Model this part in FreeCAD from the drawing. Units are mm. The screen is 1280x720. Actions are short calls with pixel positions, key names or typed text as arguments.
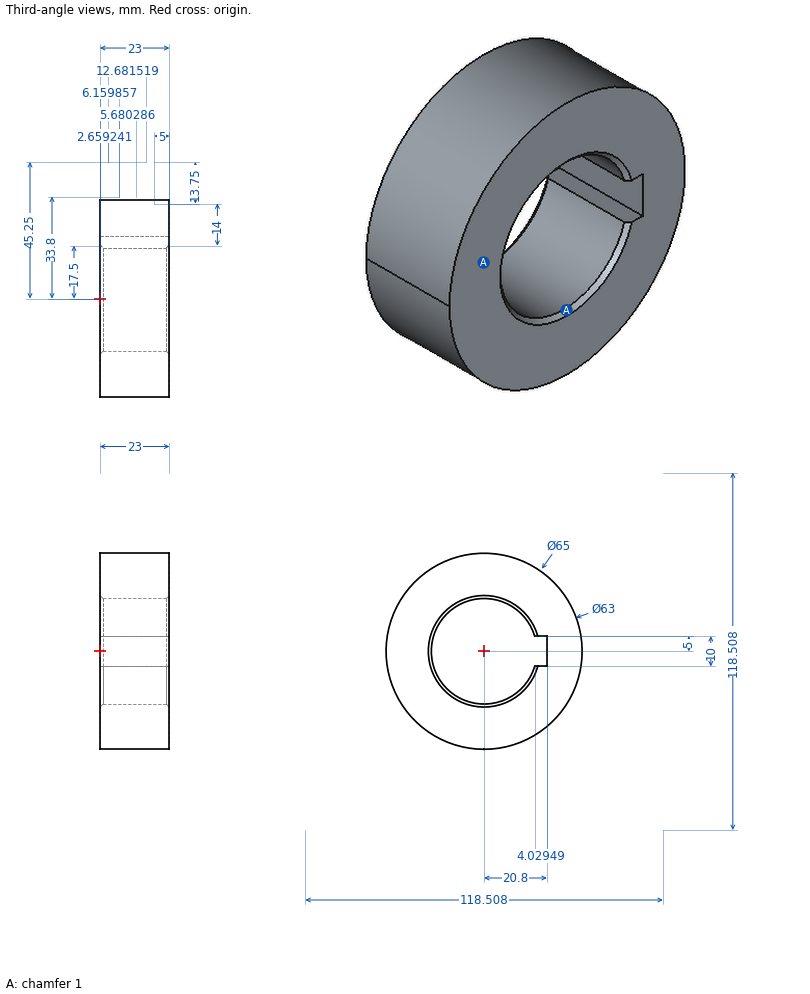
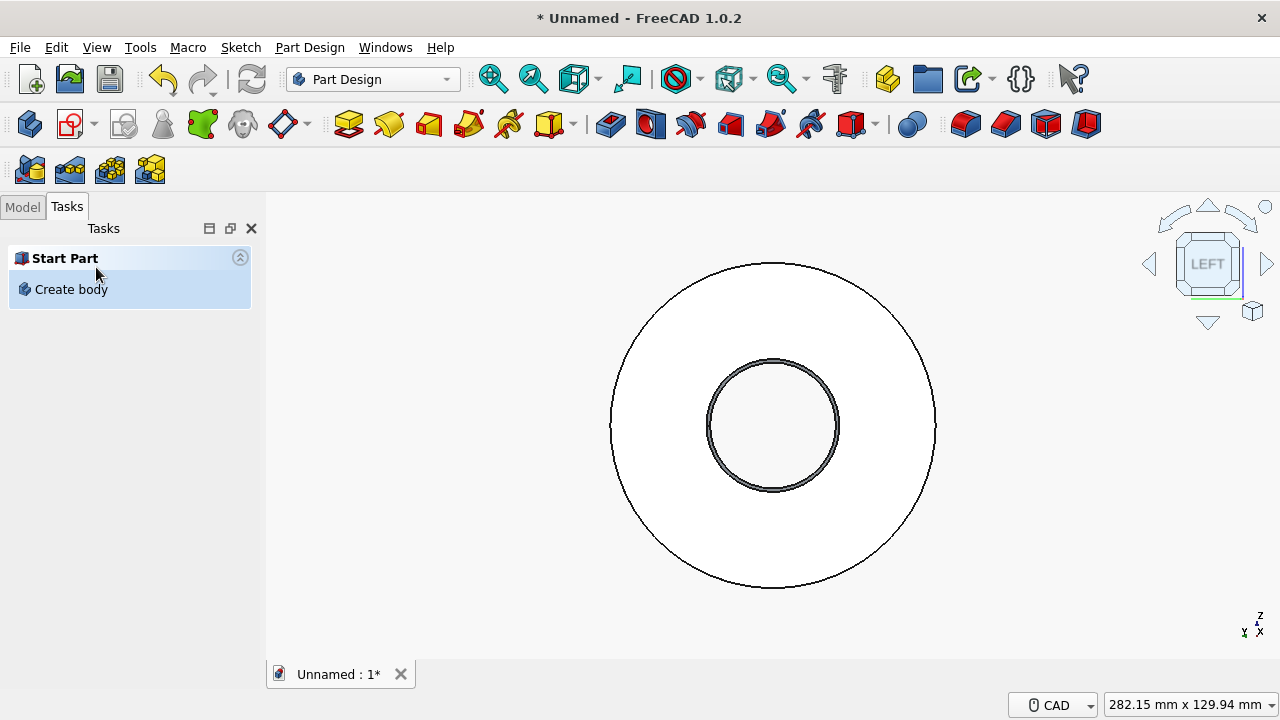
click(70, 124)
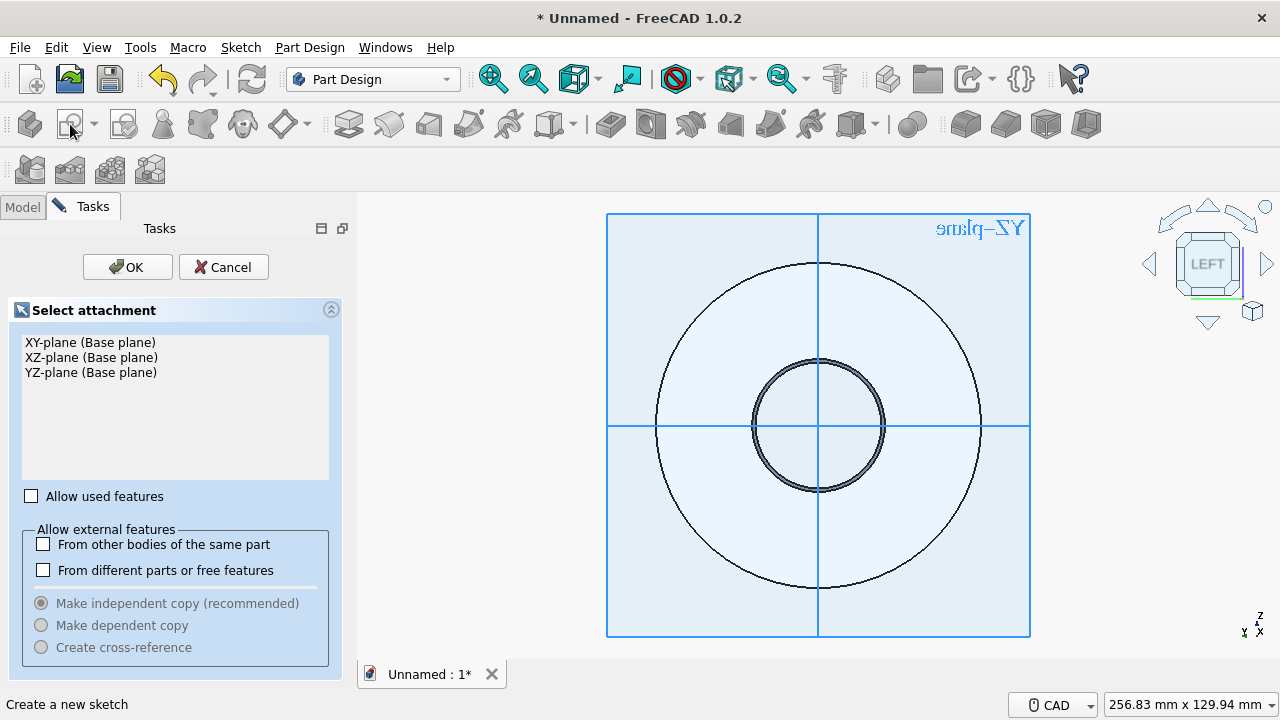
click(82, 372)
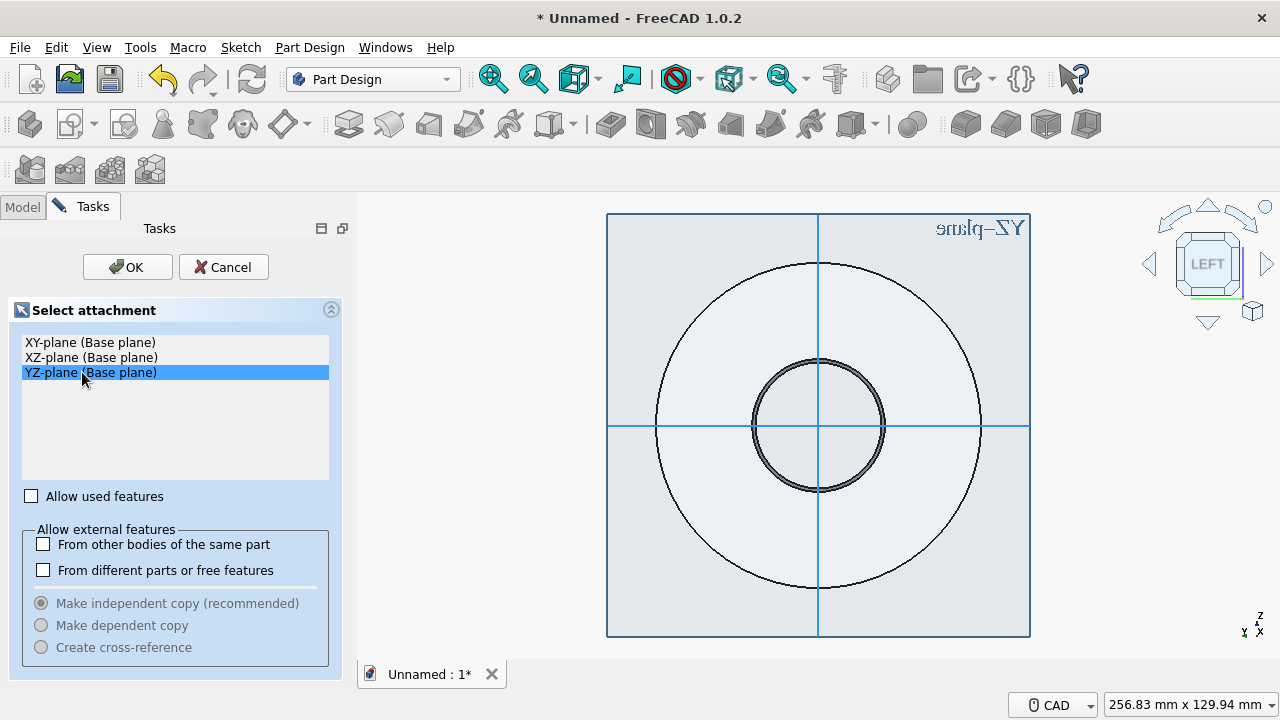
click(128, 267)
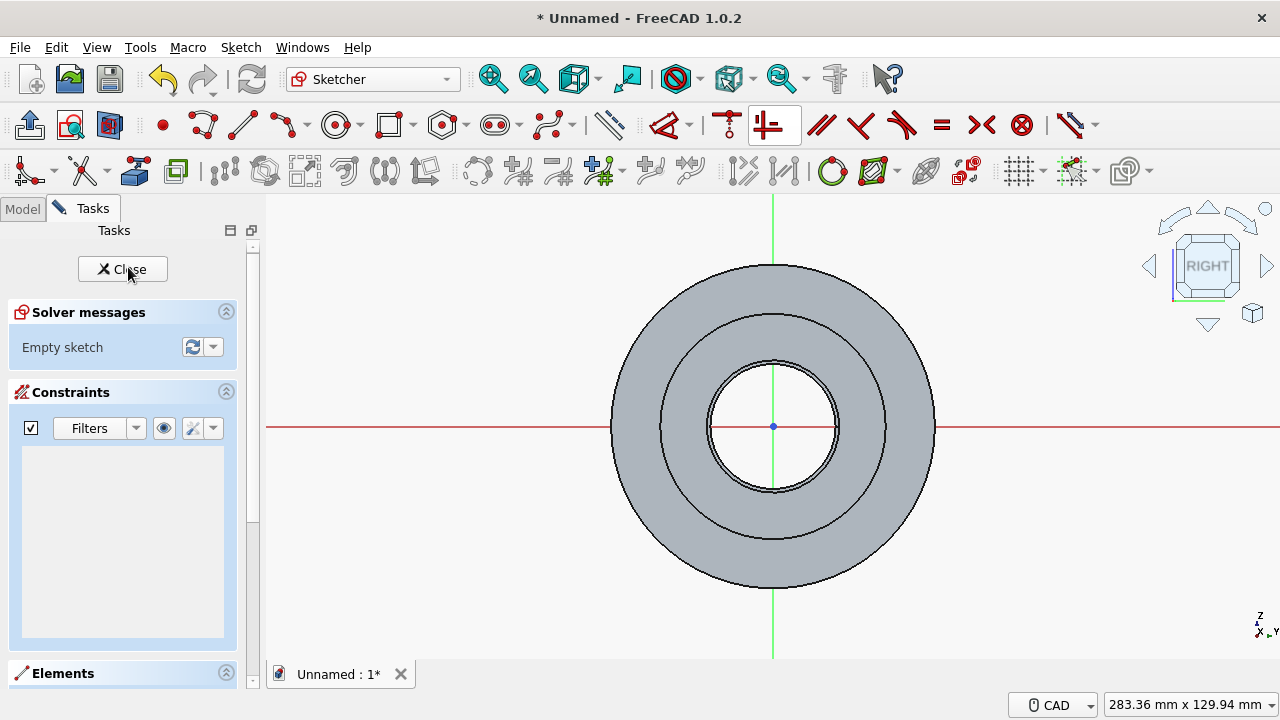
key(q)
key(s)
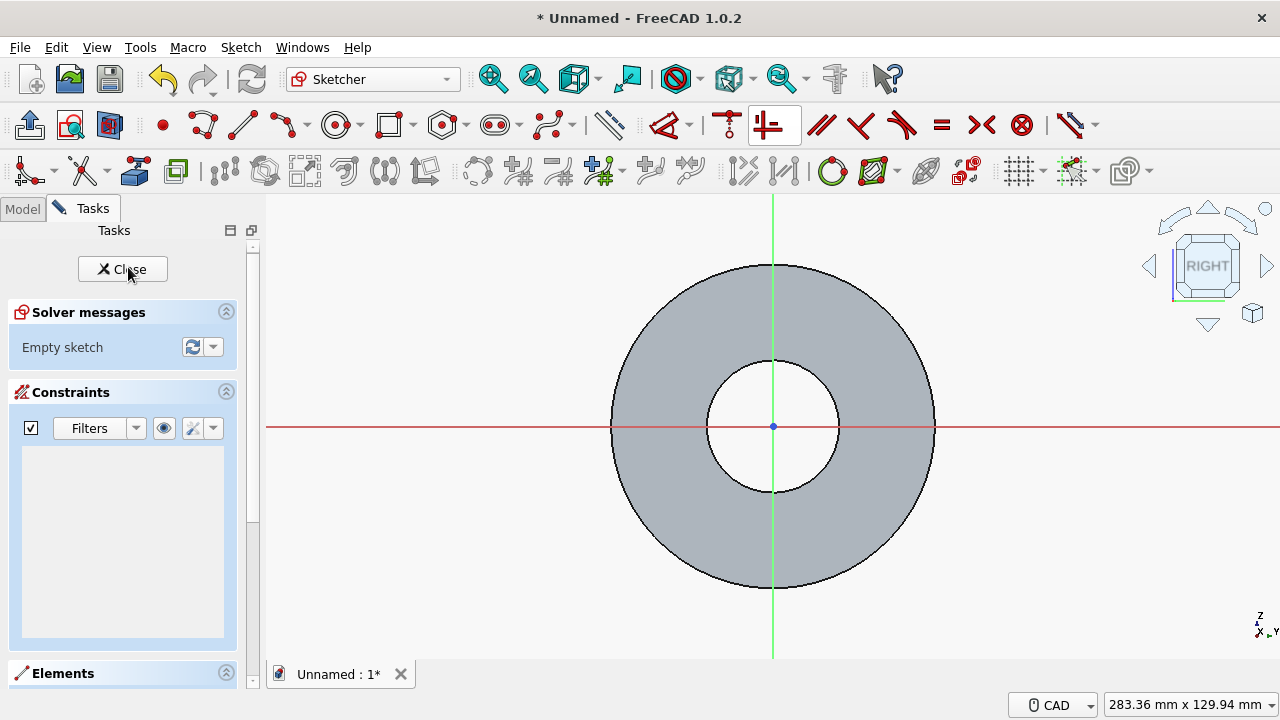
scroll(827, 426, up, 10)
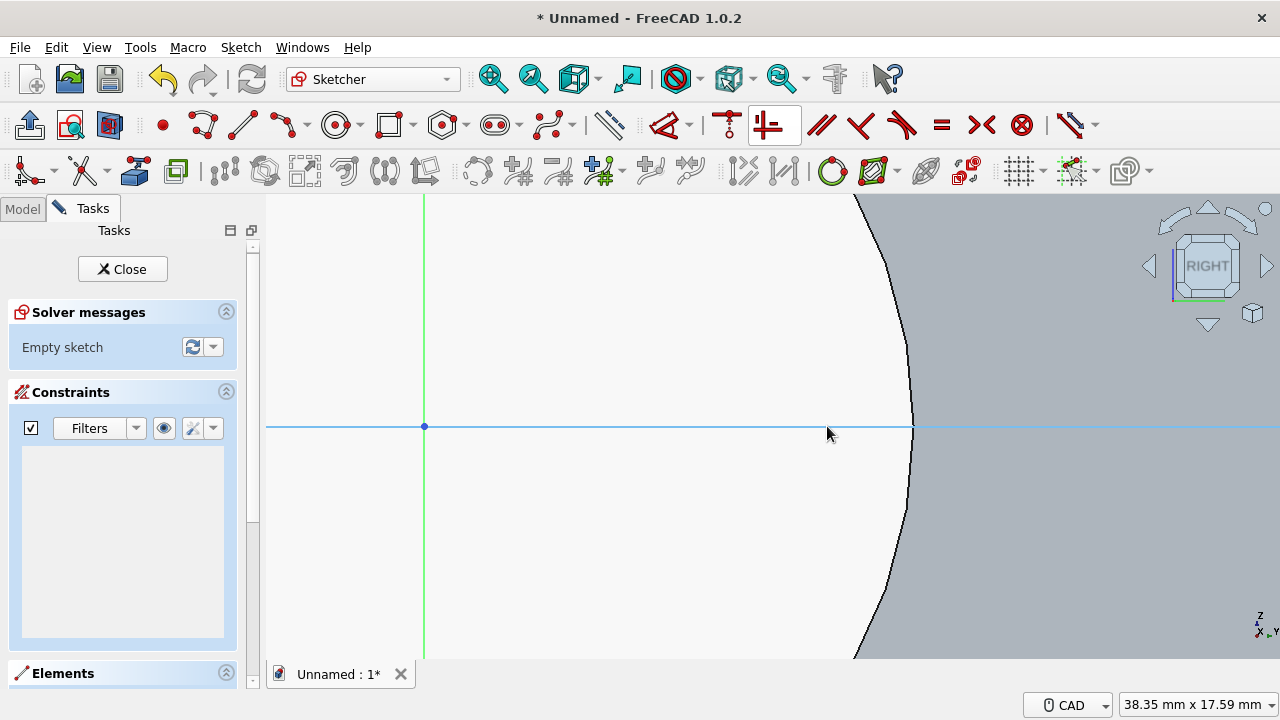
key(g)
key(r)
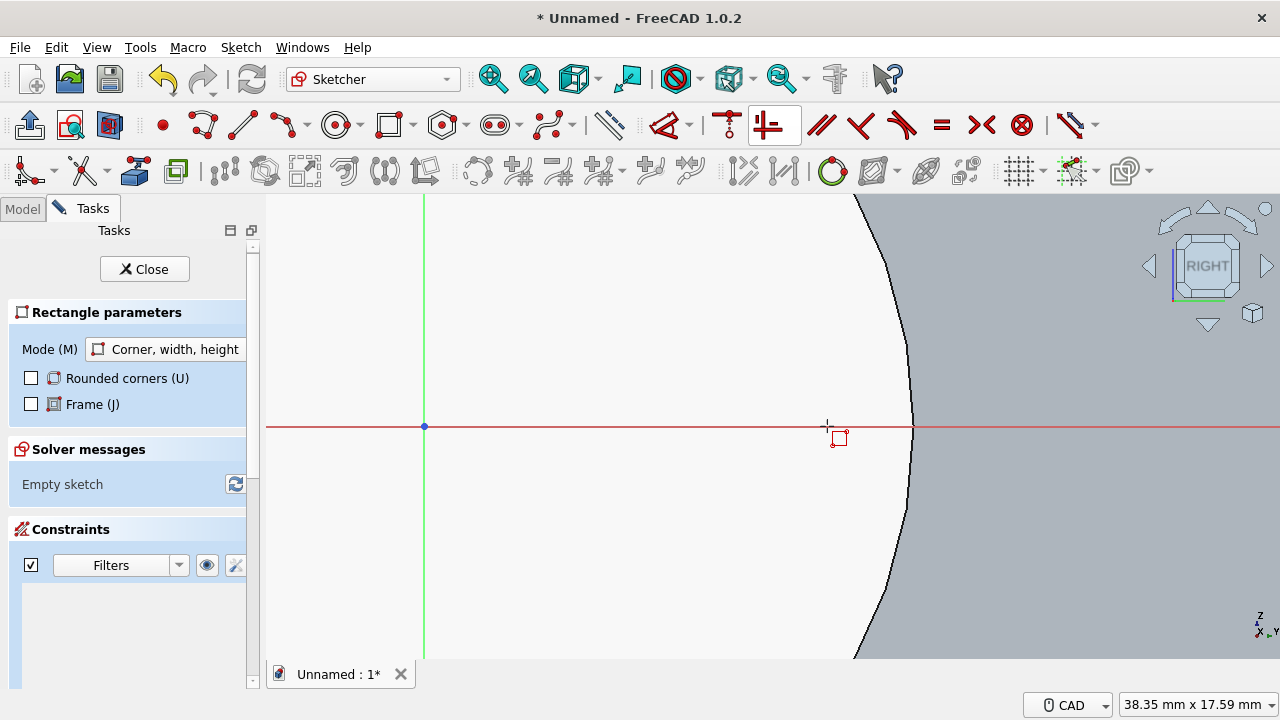
click(868, 294)
move(974, 559)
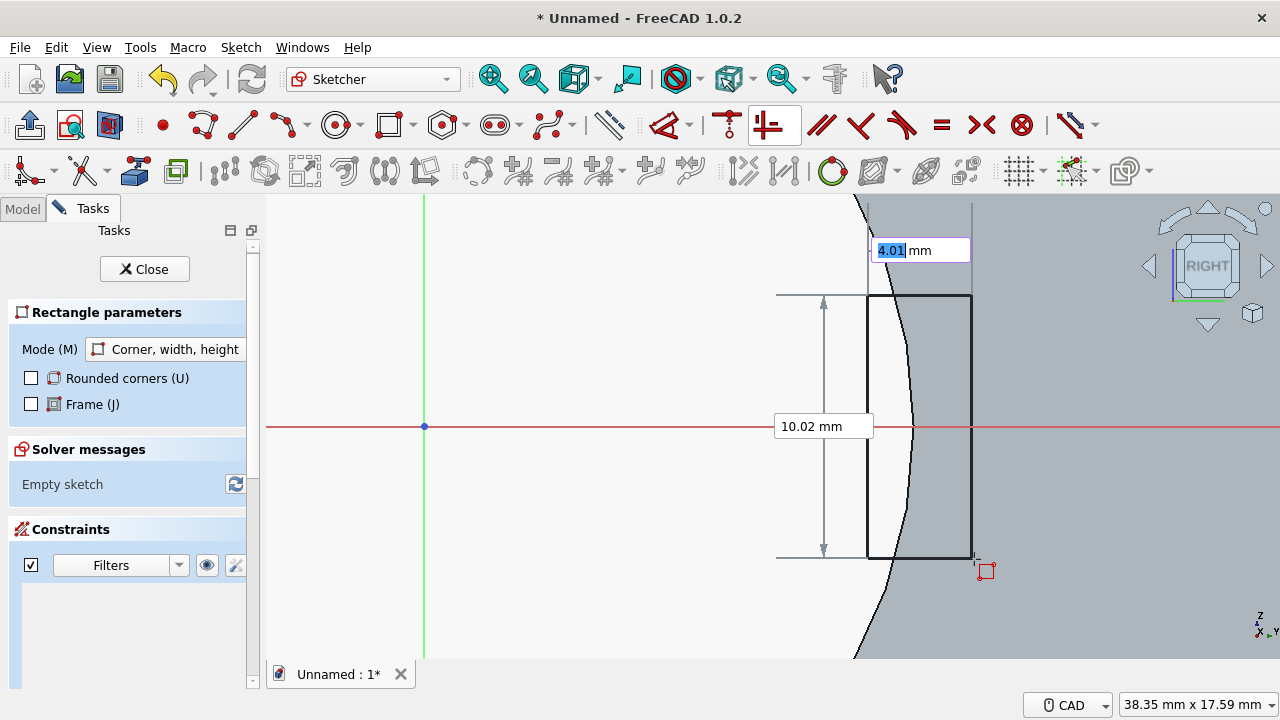
text(4.02949)
key(Tab)
text(10)
key(Return)
key(Escape)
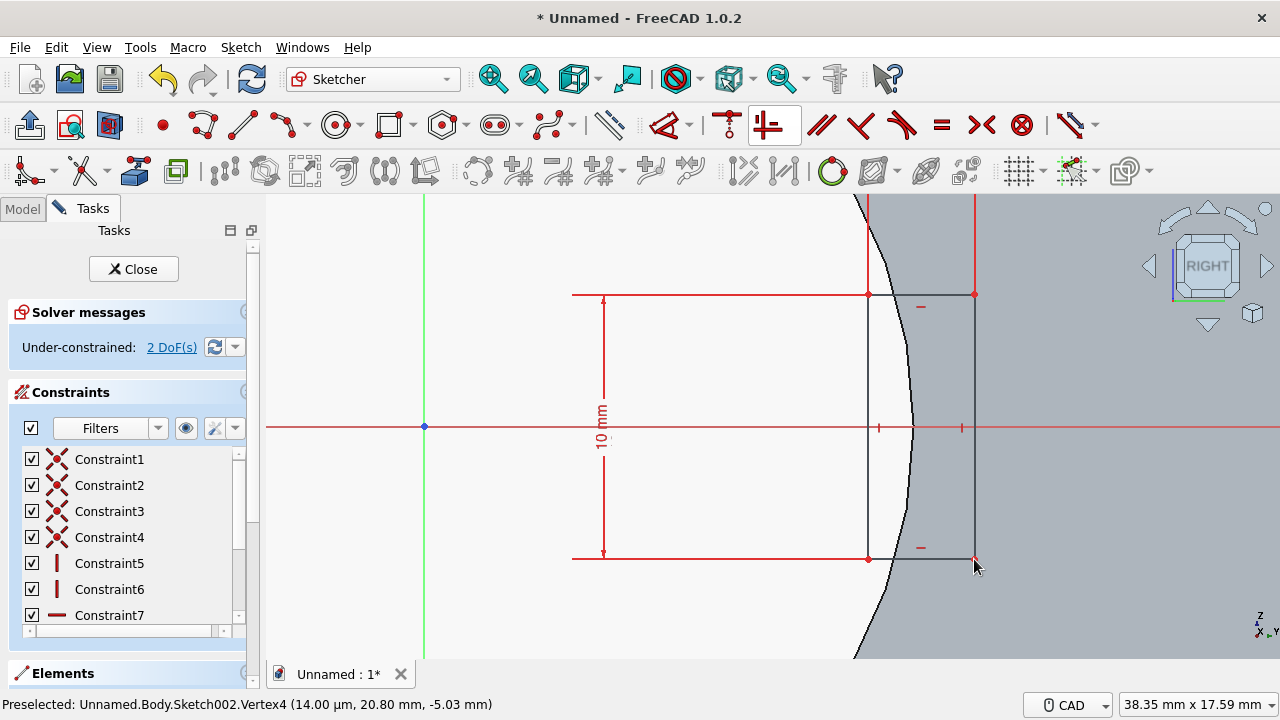
key(d)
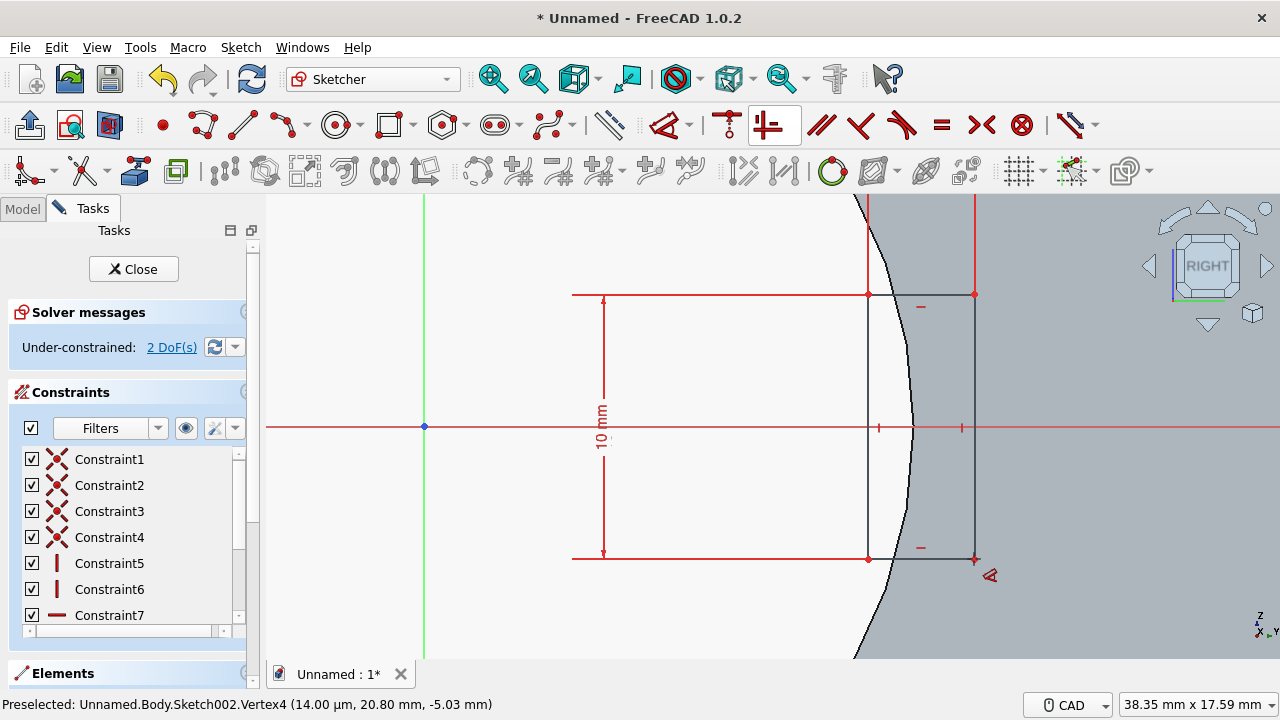
click(868, 295)
click(390, 361)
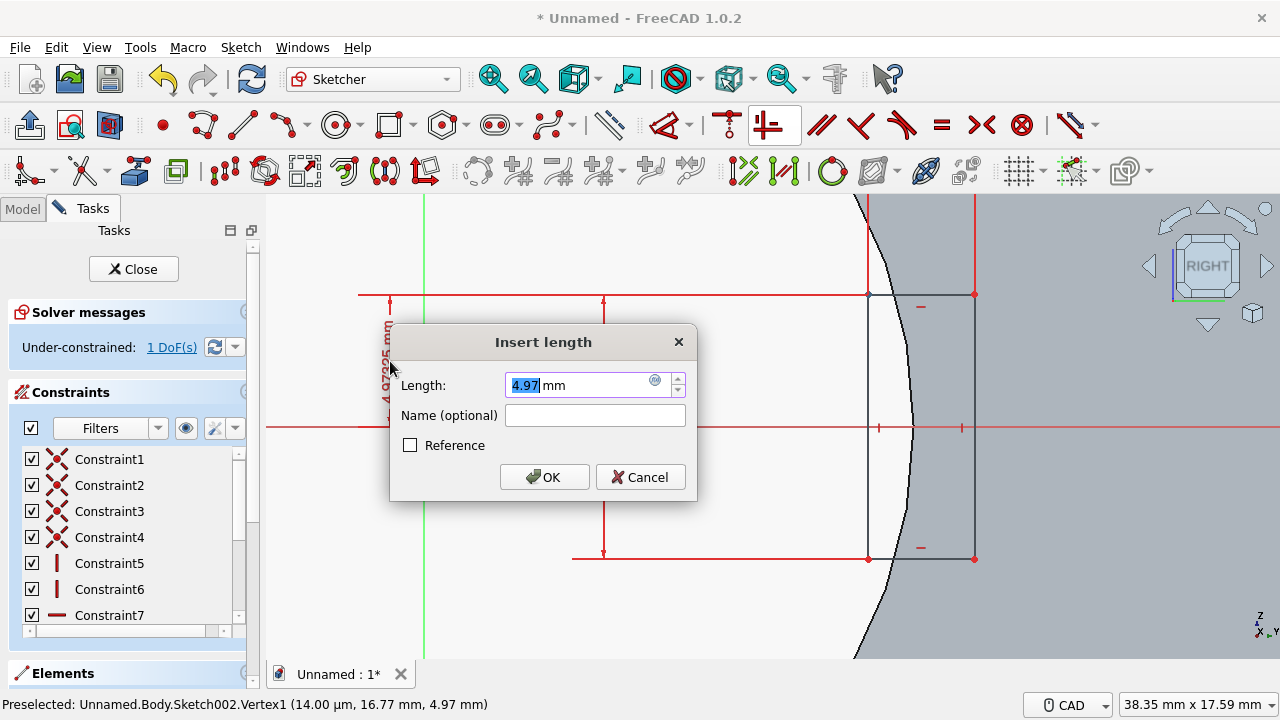
text(5)
key(Return)